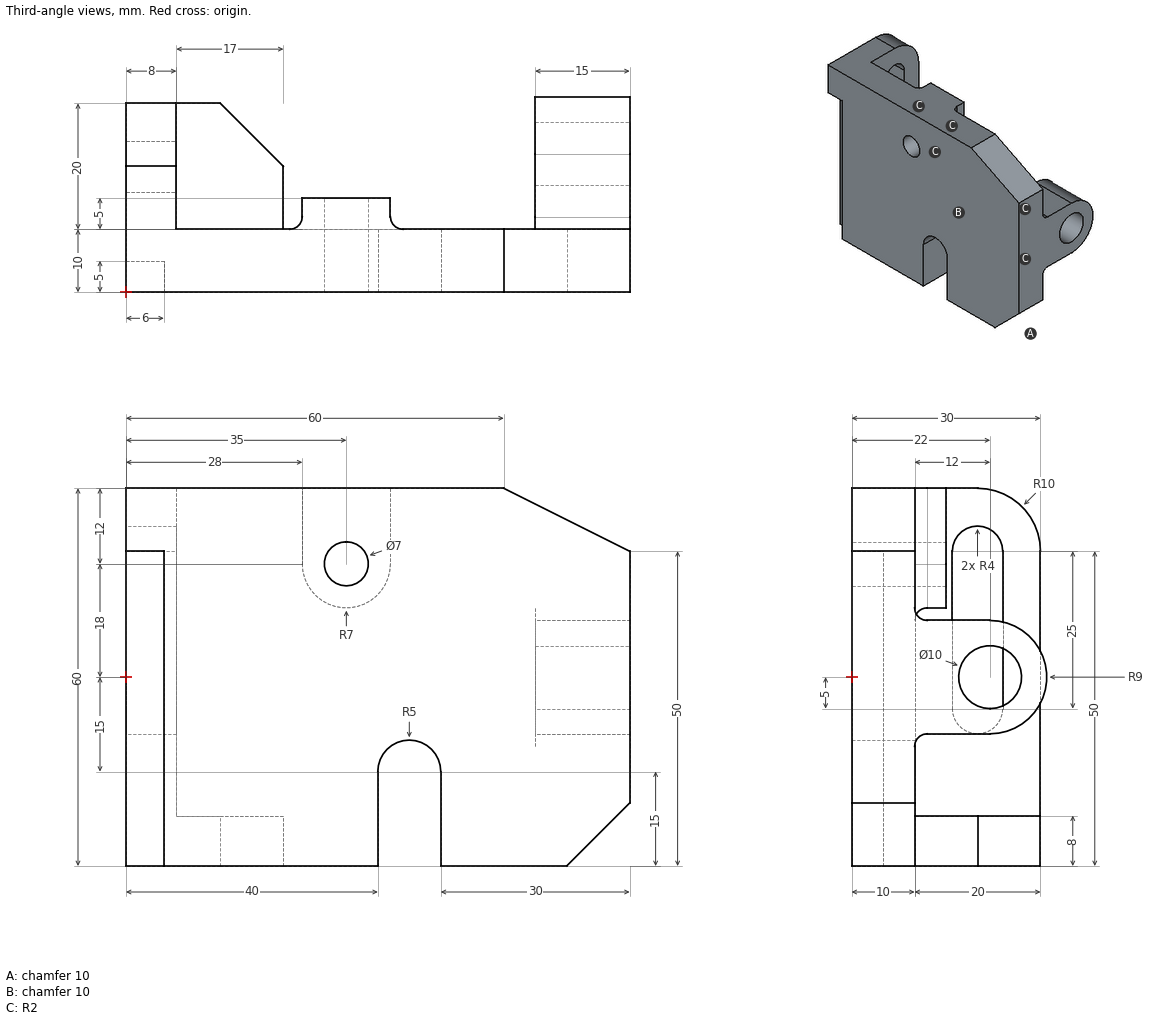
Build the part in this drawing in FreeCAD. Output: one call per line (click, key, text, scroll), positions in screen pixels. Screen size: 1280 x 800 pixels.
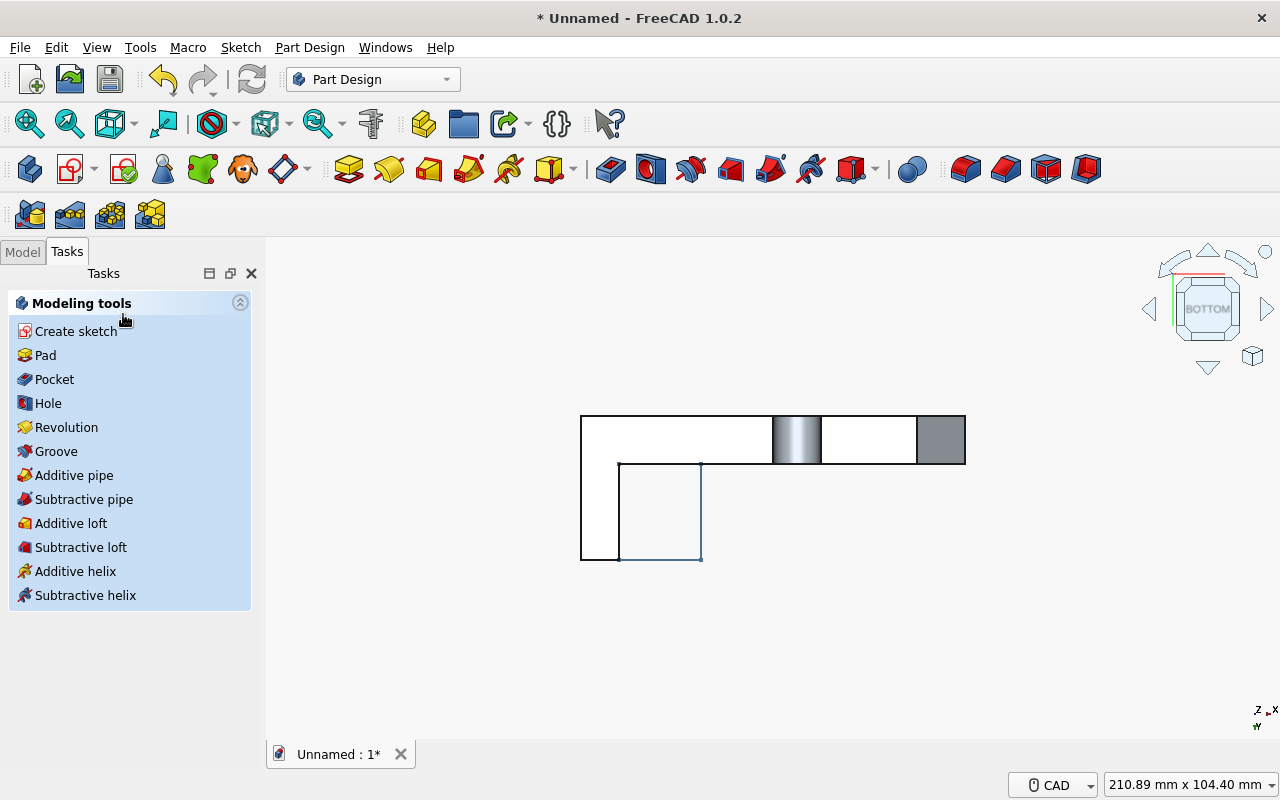
click(350, 170)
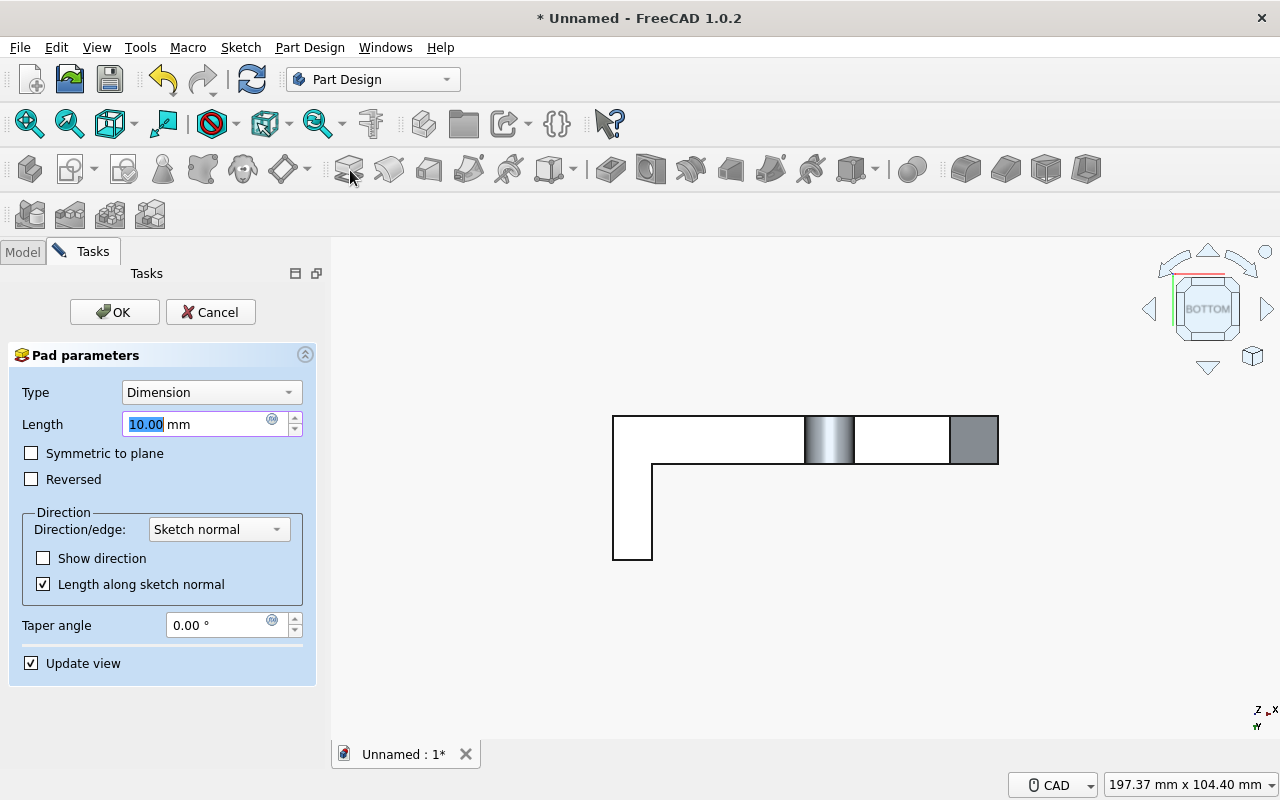
text(8)
key(Tab)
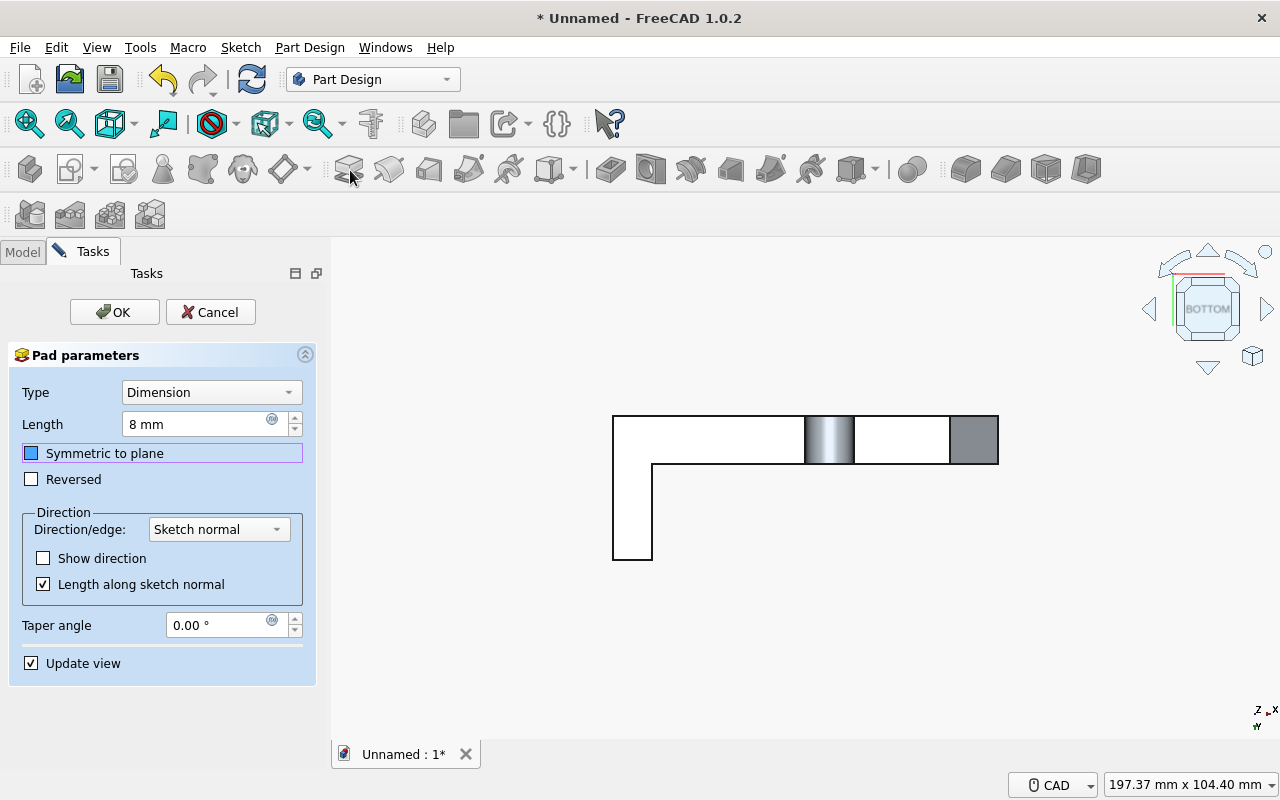
click(30, 479)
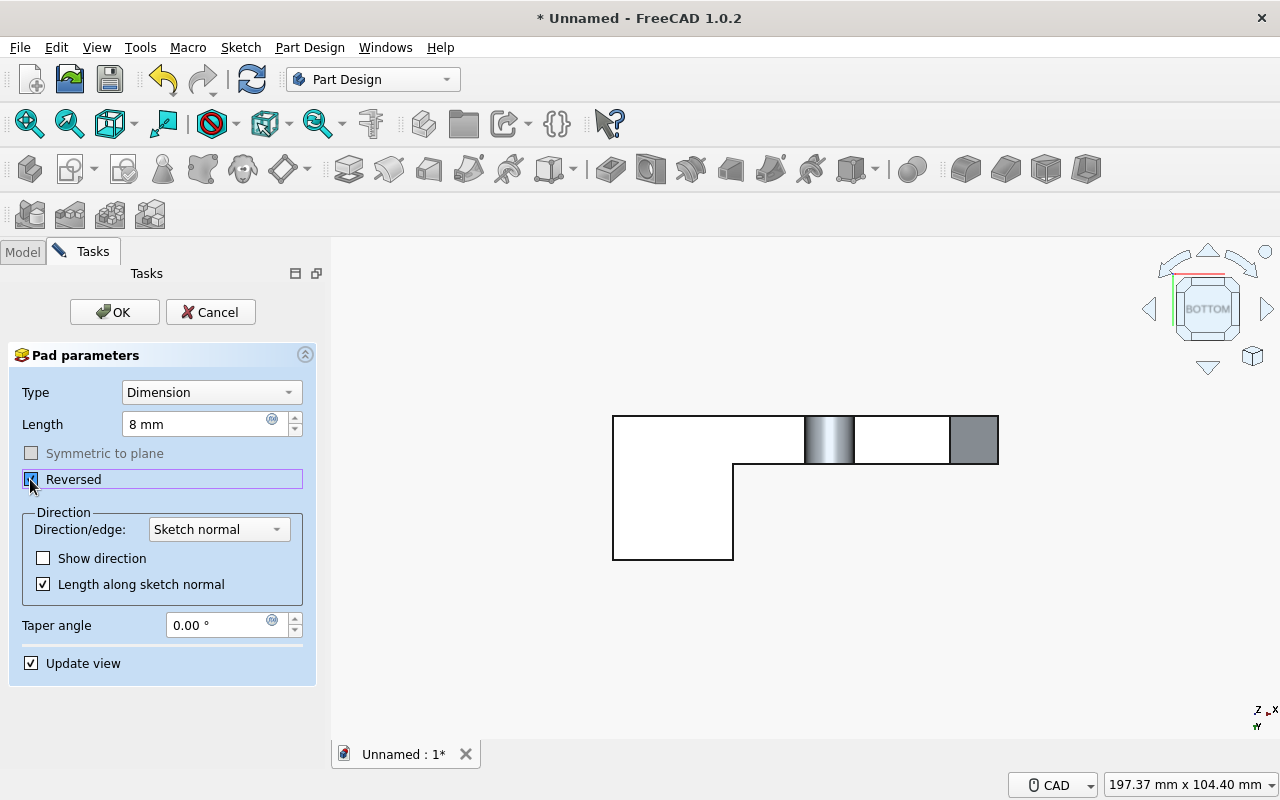
click(115, 312)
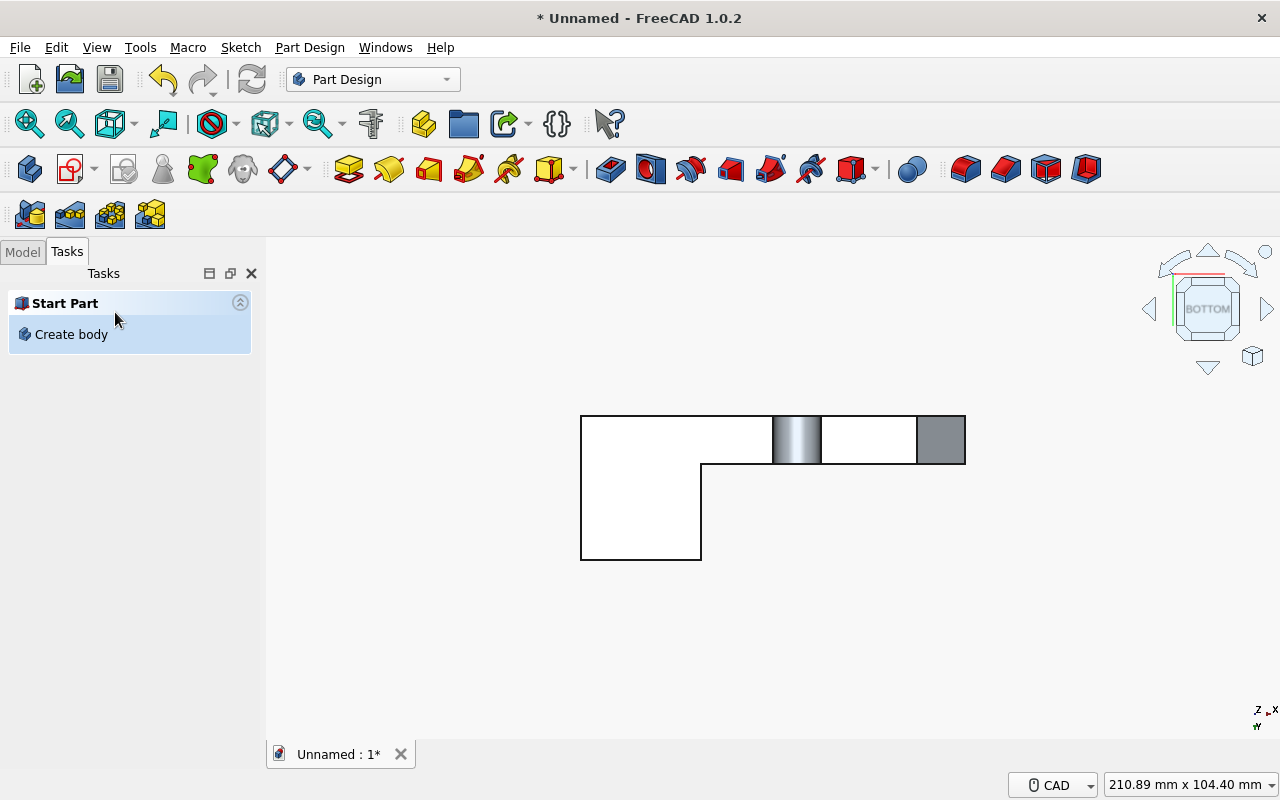
click(30, 124)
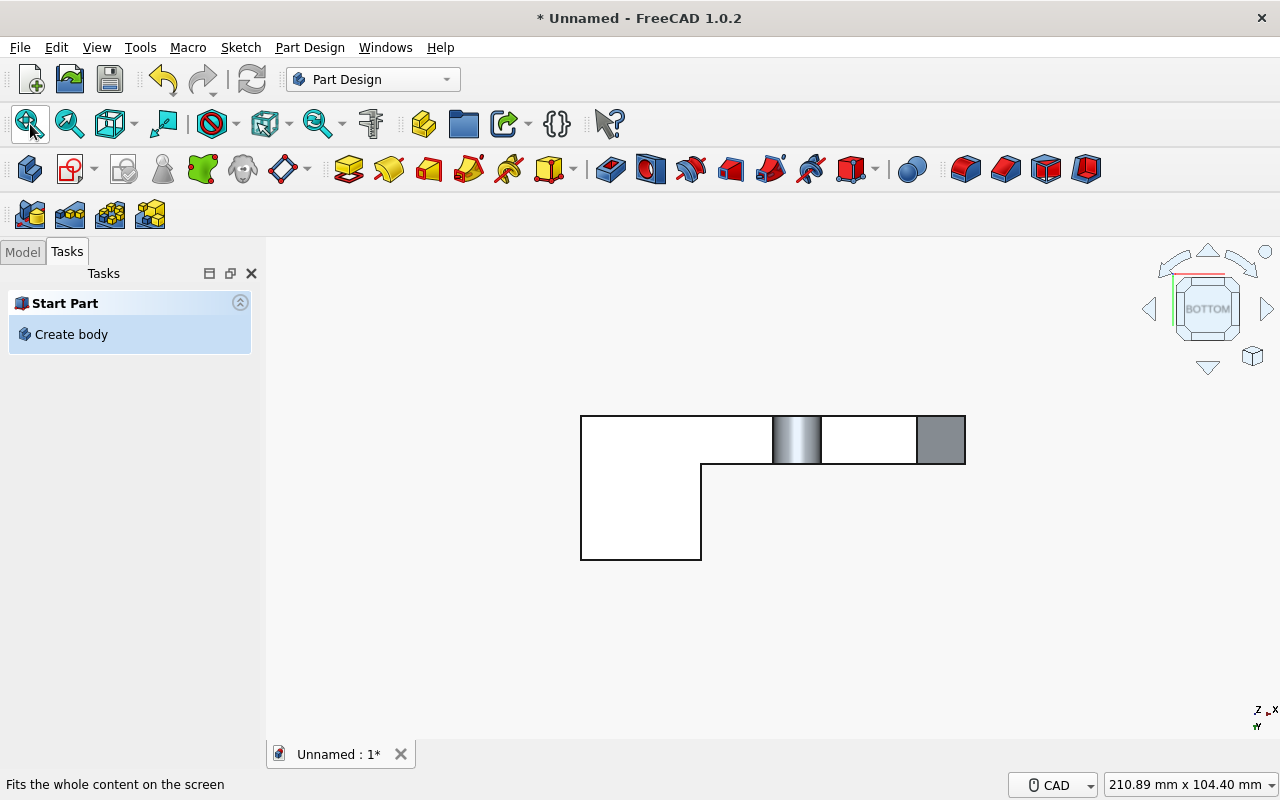
key(0)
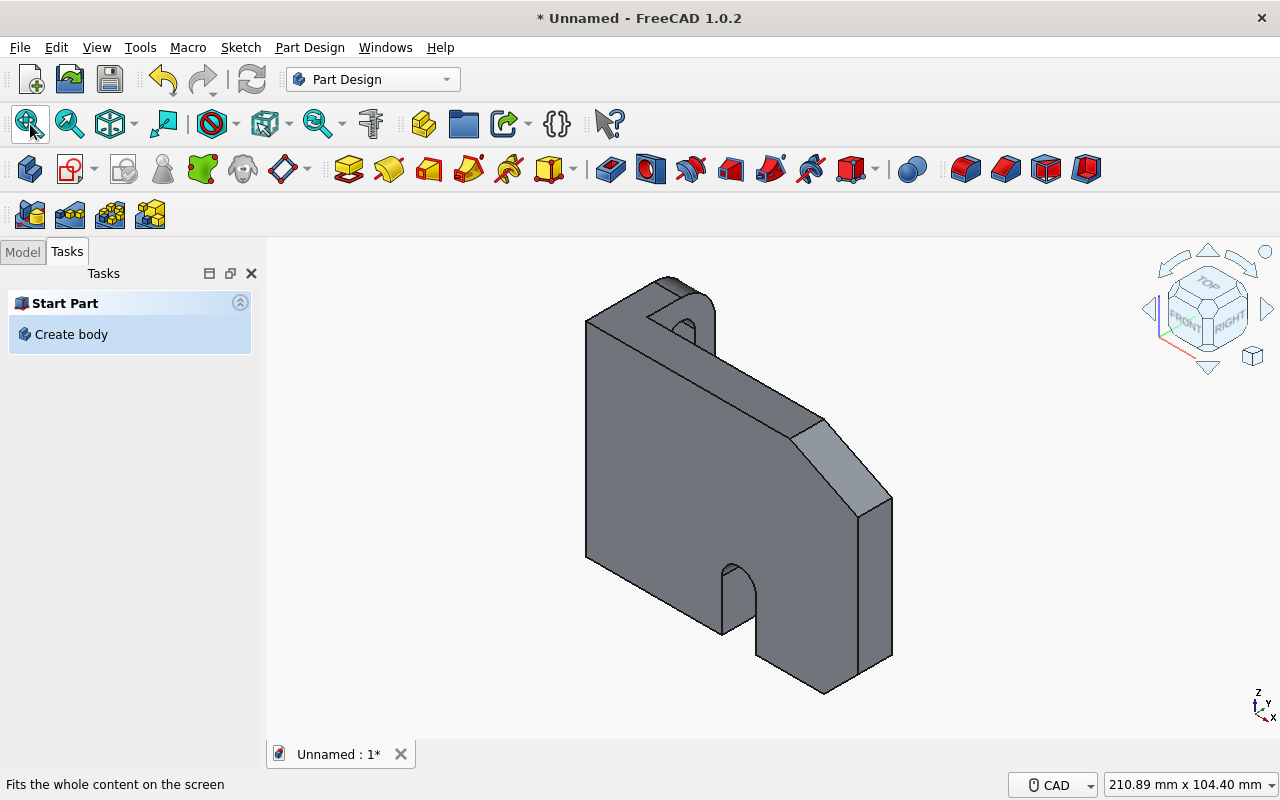
key(2)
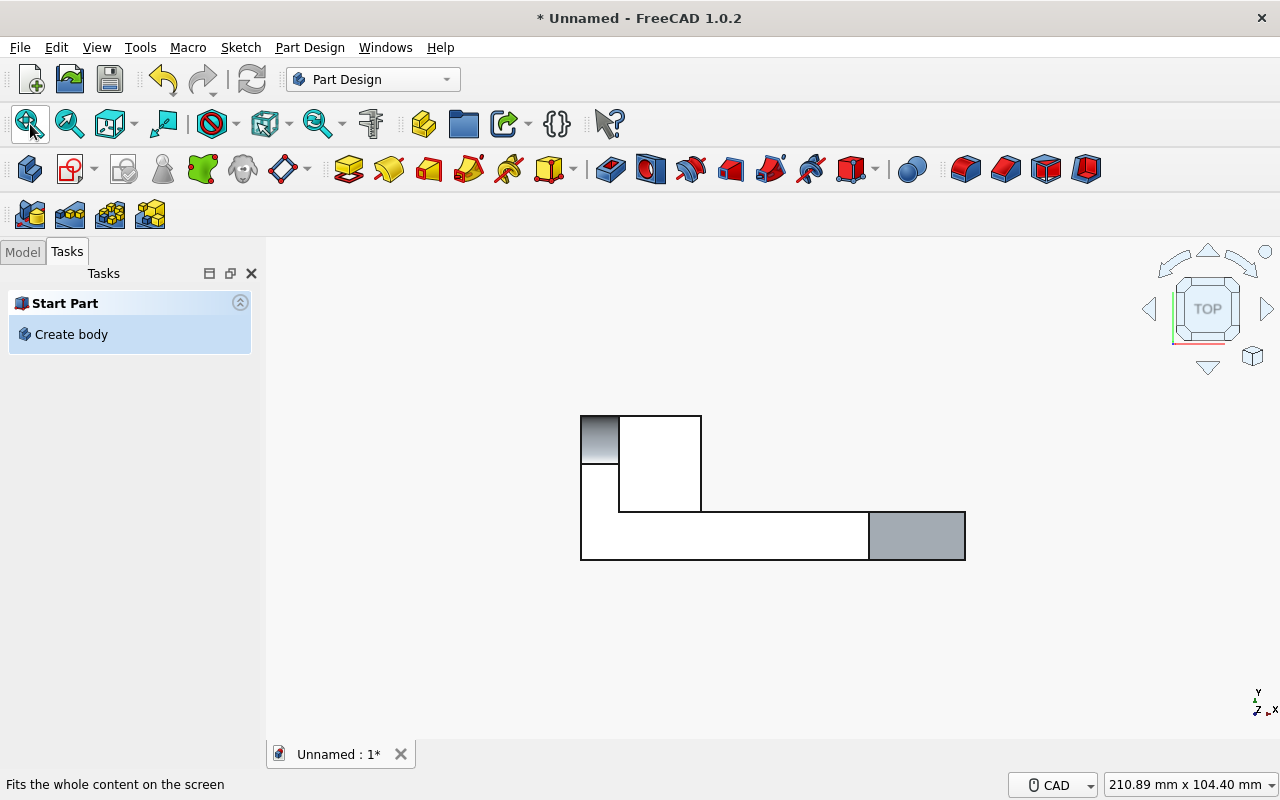
click(30, 124)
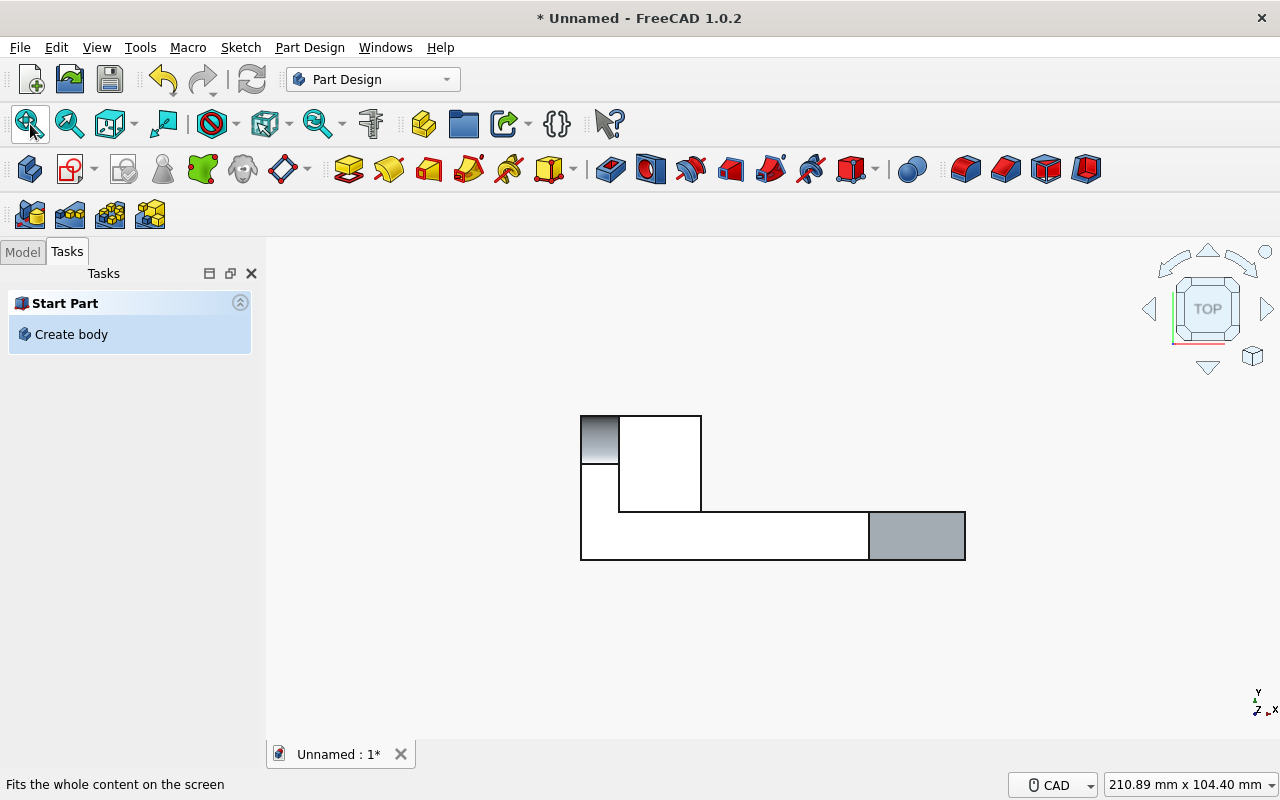
key(1)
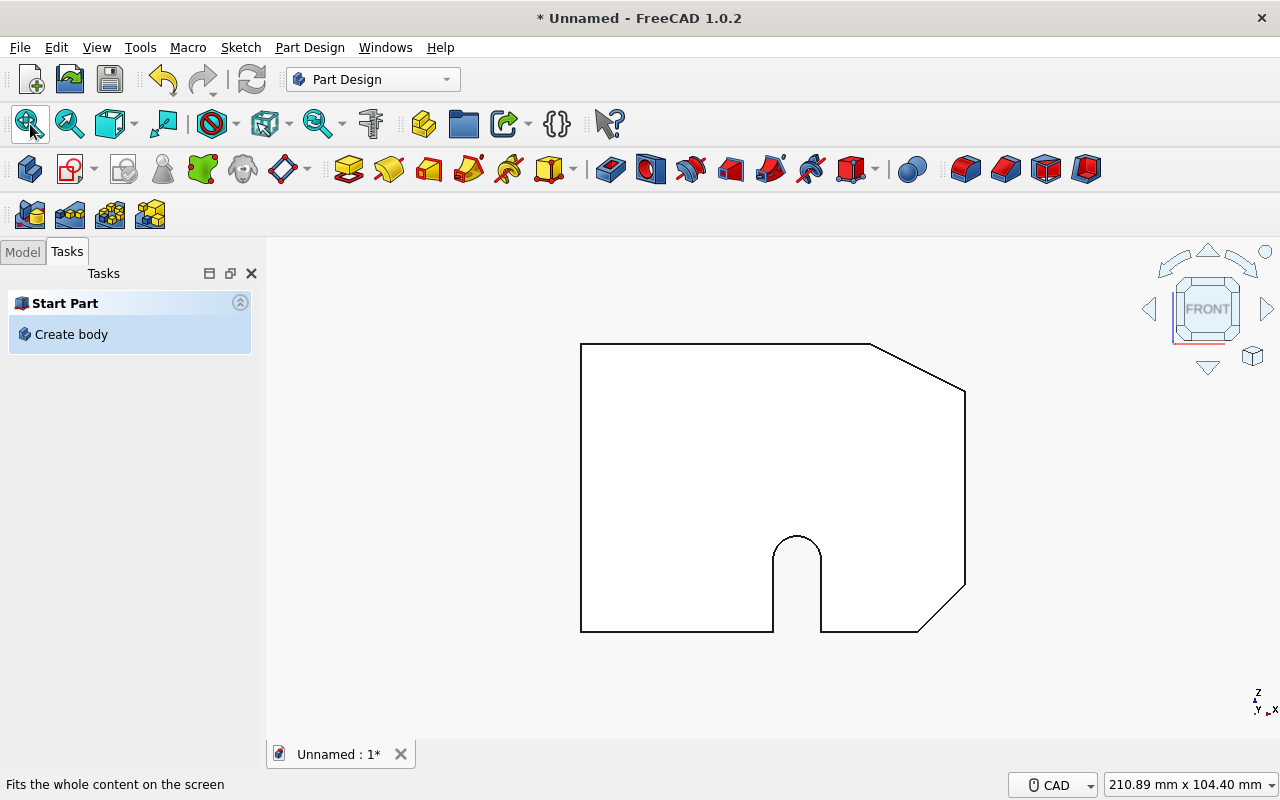
key(3)